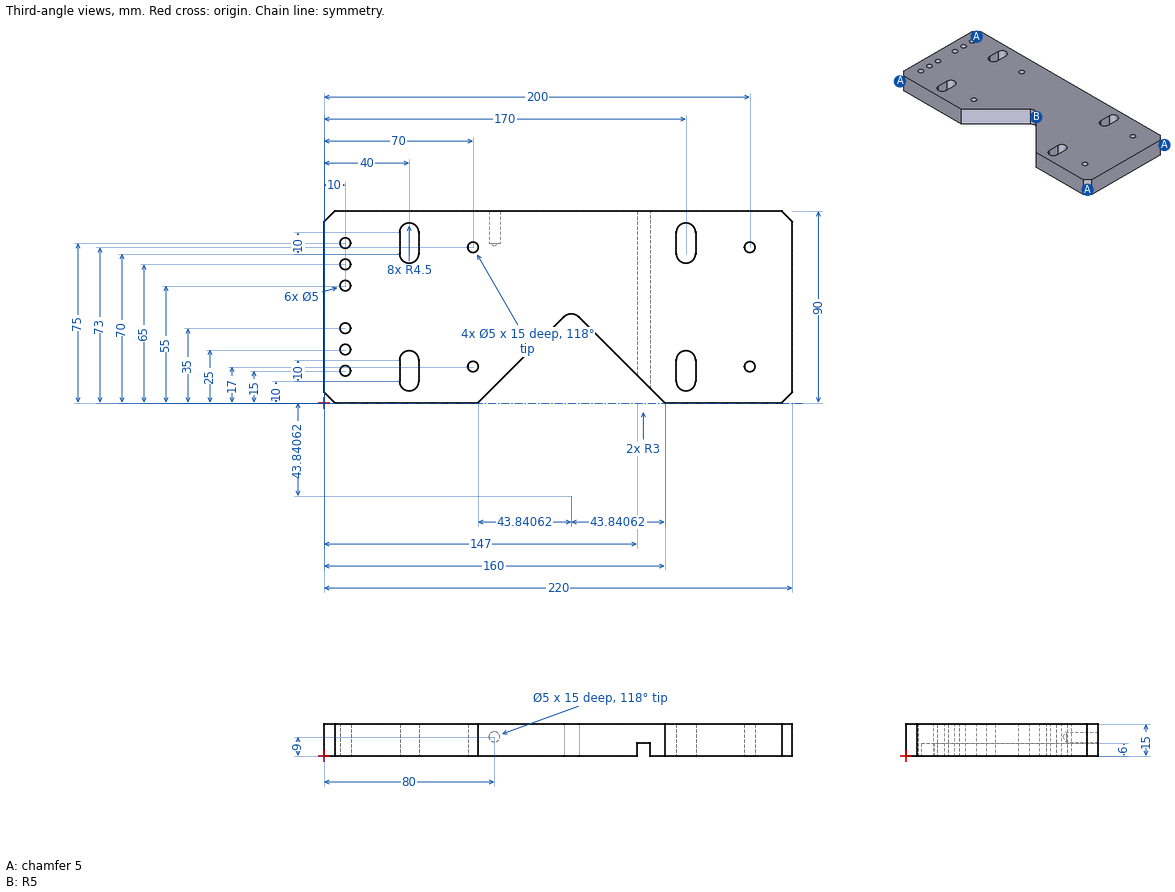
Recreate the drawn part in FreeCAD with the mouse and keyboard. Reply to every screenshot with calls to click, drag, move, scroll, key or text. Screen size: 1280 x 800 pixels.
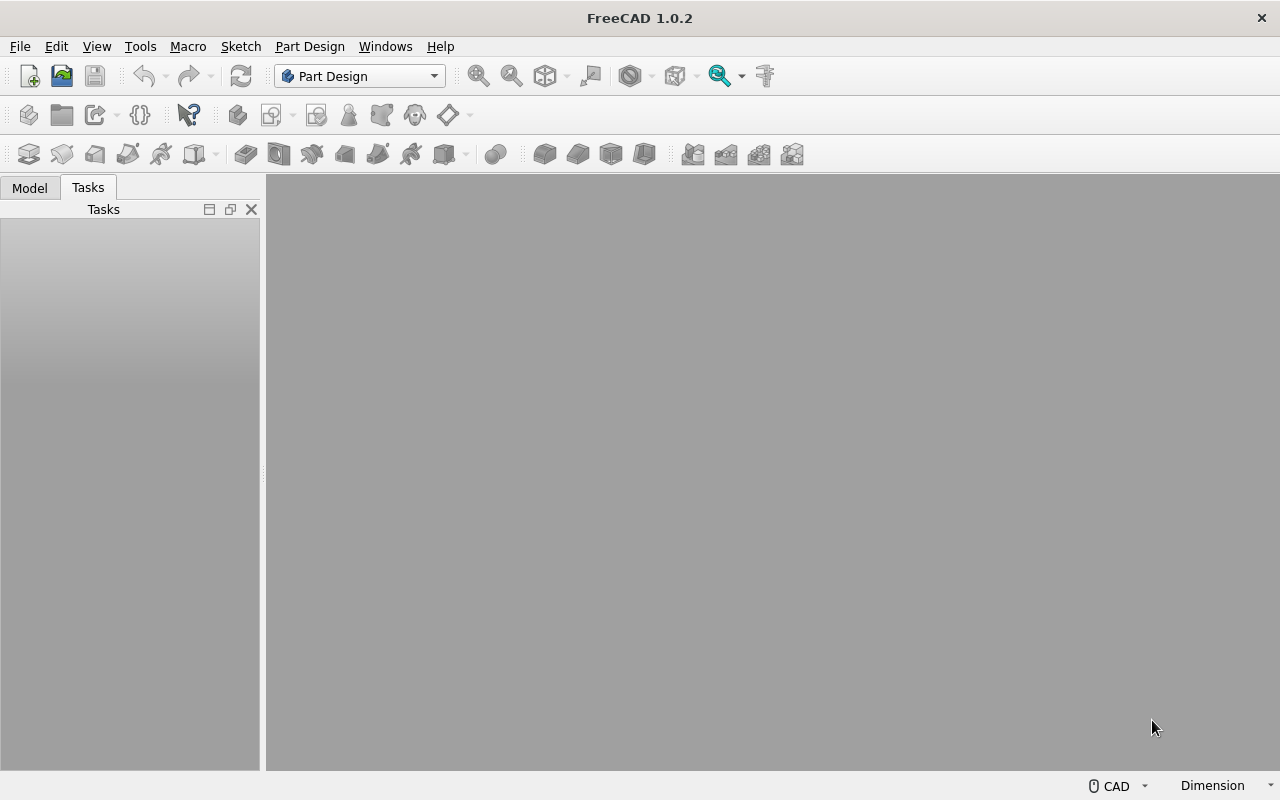
click(29, 76)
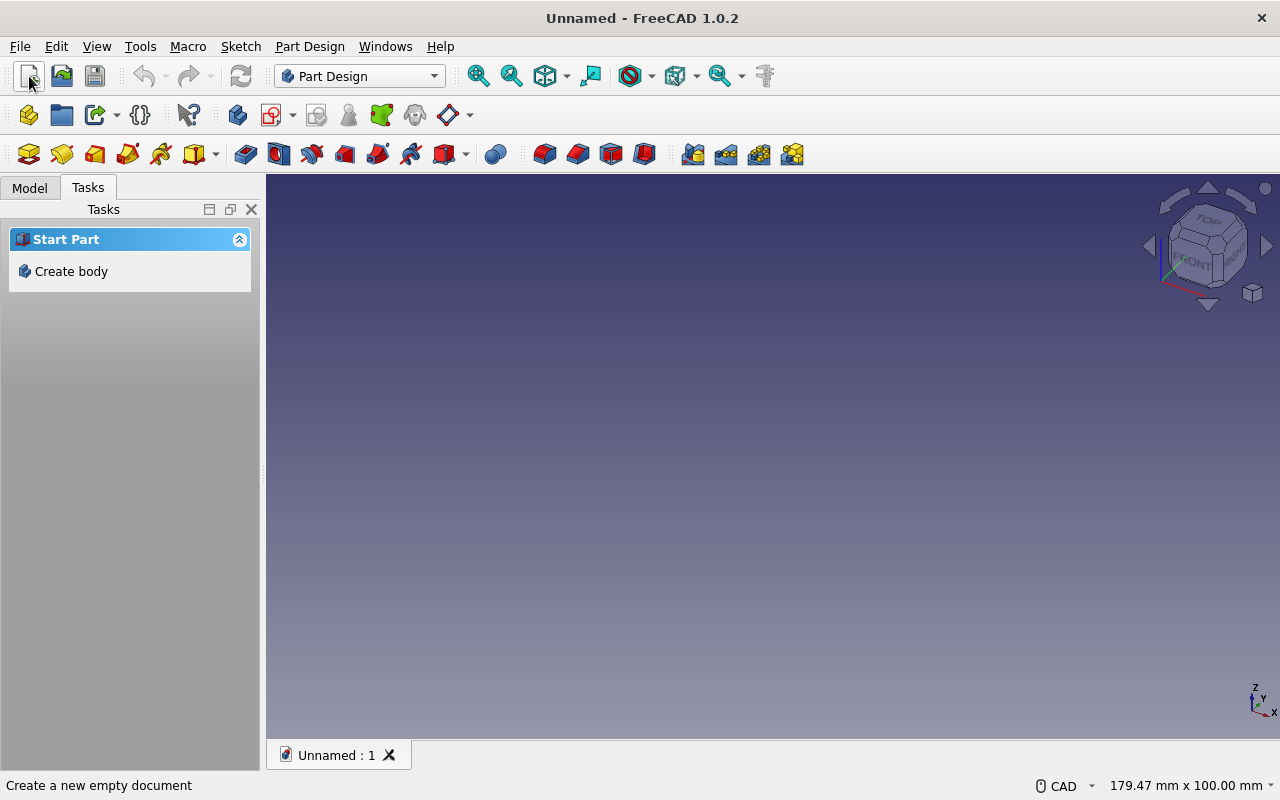
click(270, 116)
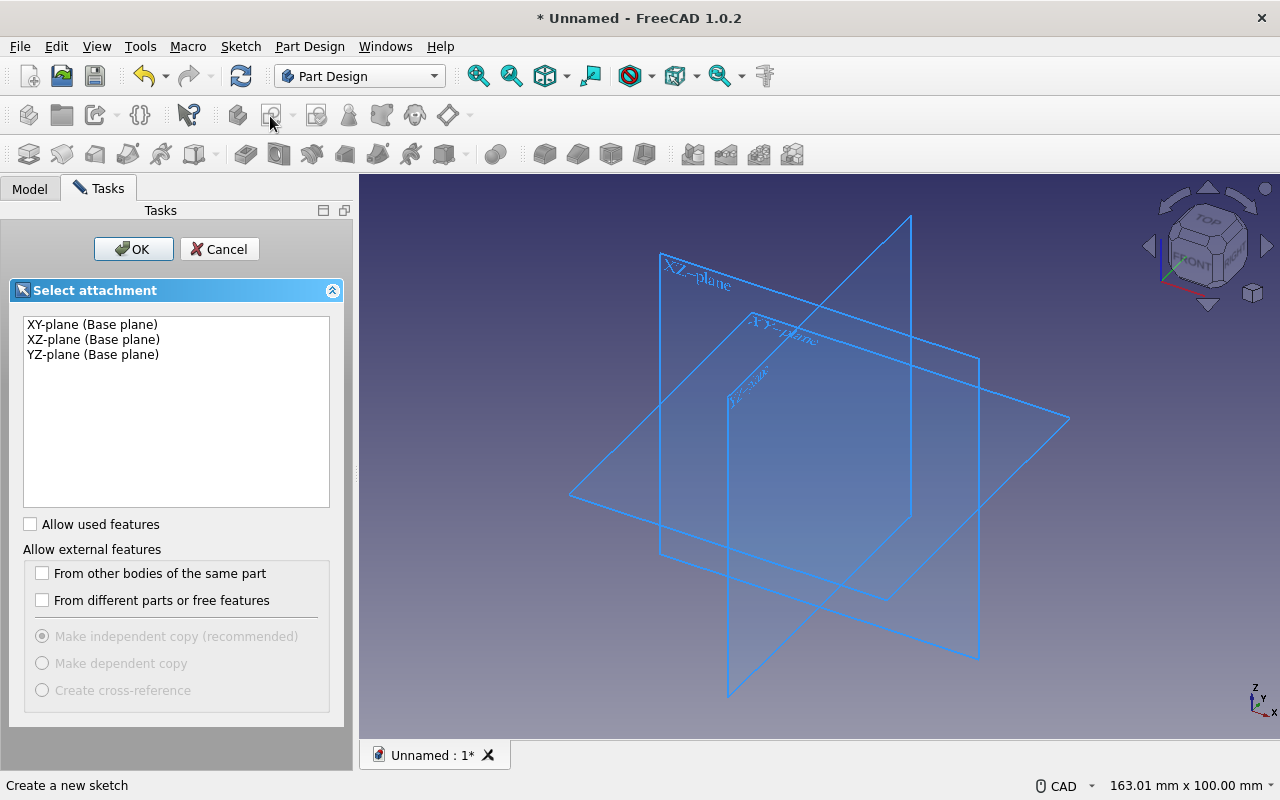
click(84, 324)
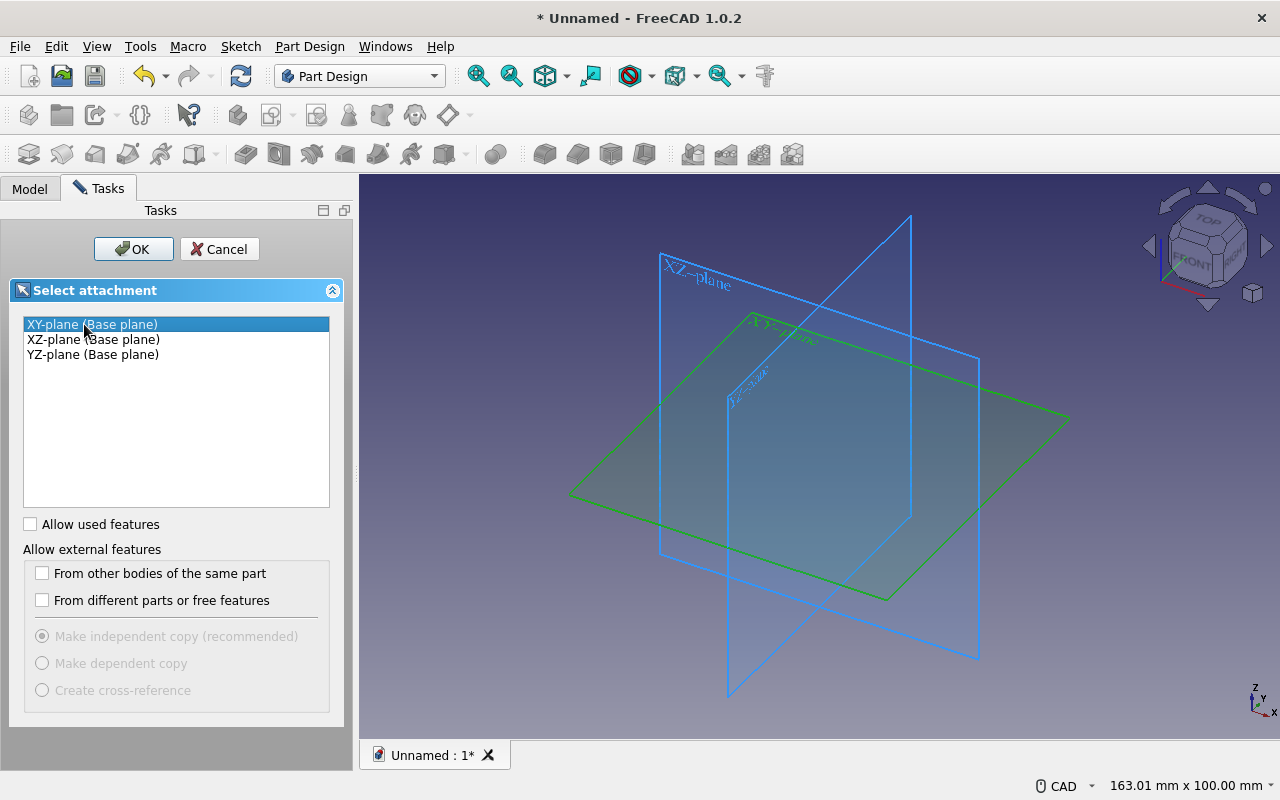
click(134, 249)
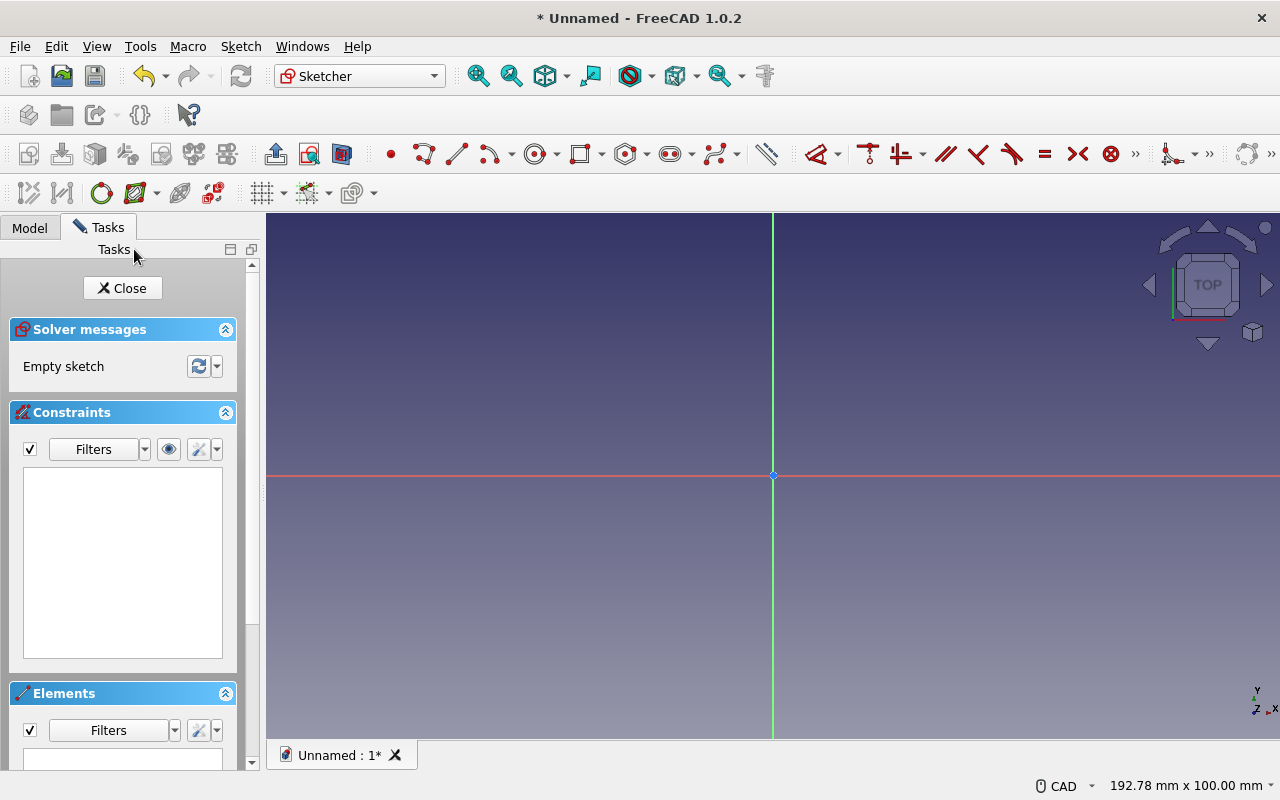
scroll(294, 669, down, 4)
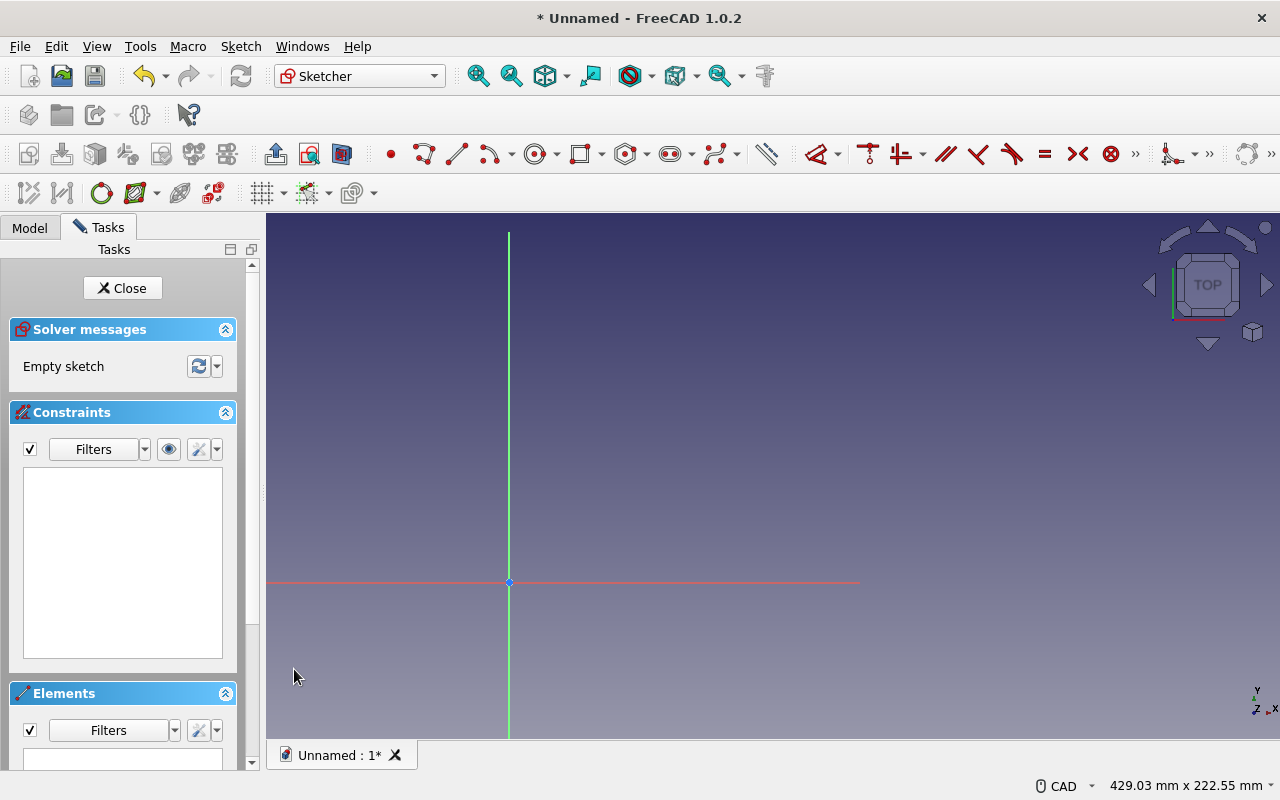
key(g)
key(r)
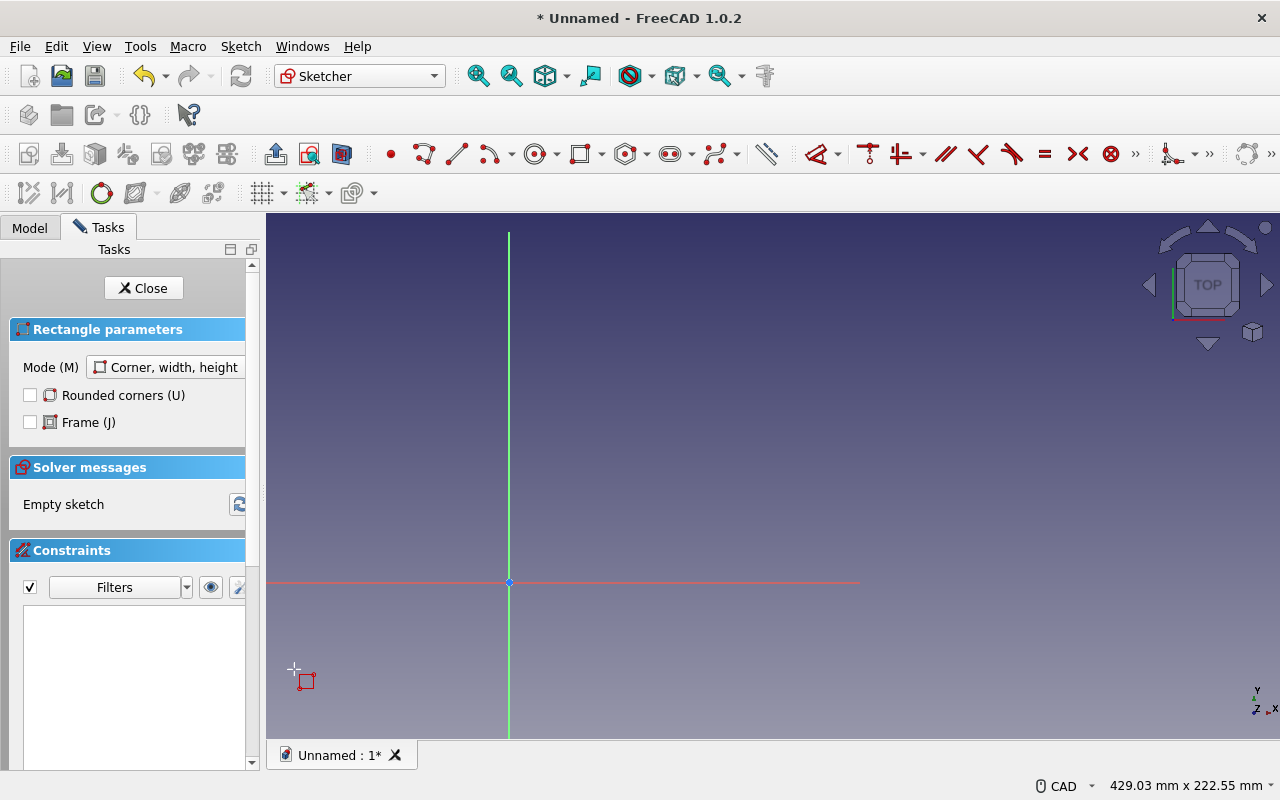
click(509, 583)
click(1029, 370)
key(Escape)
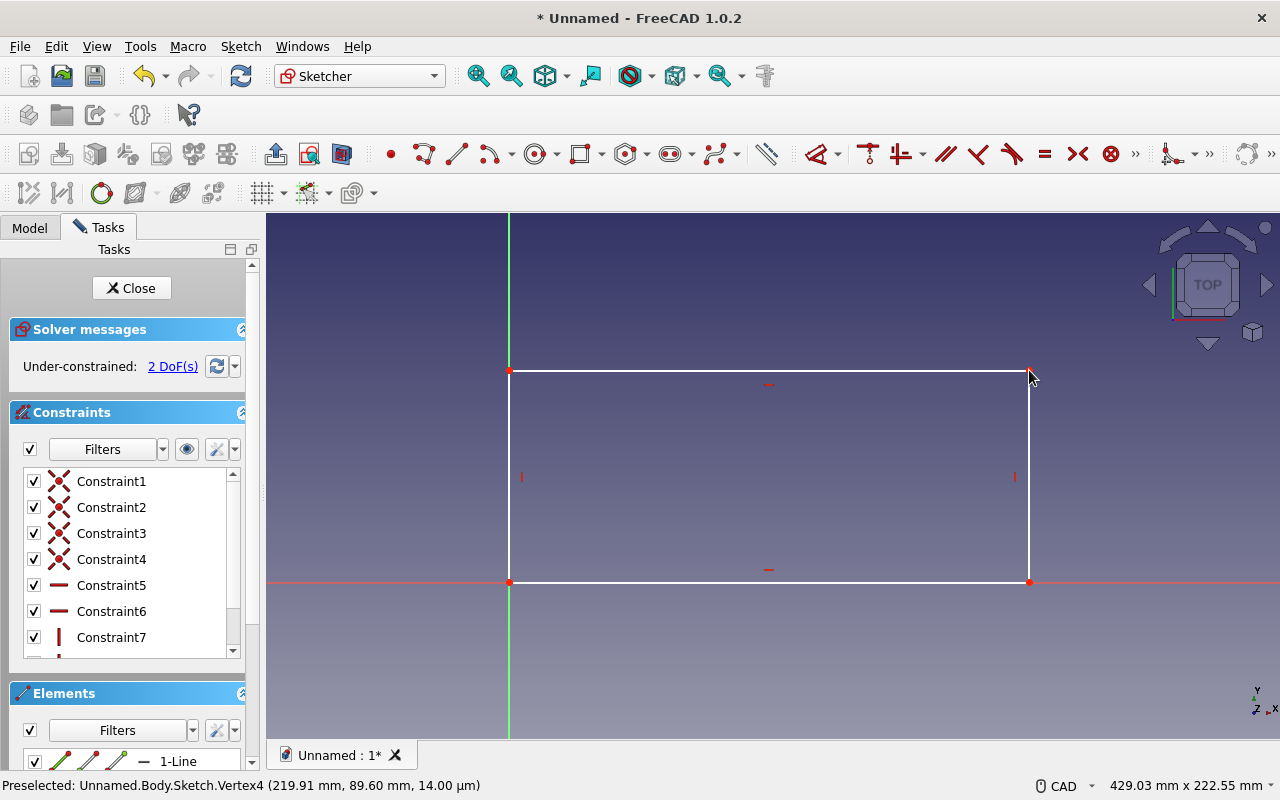
key(d)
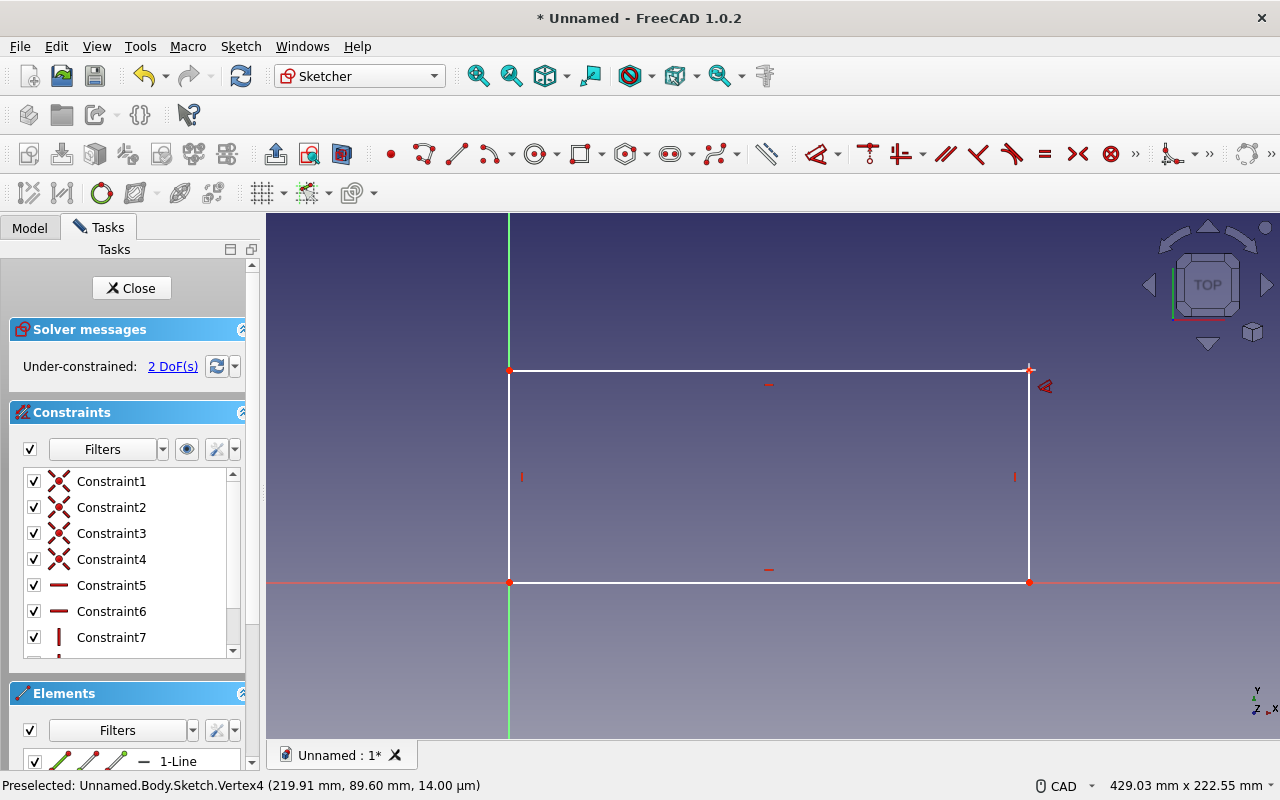
click(1029, 519)
click(1063, 477)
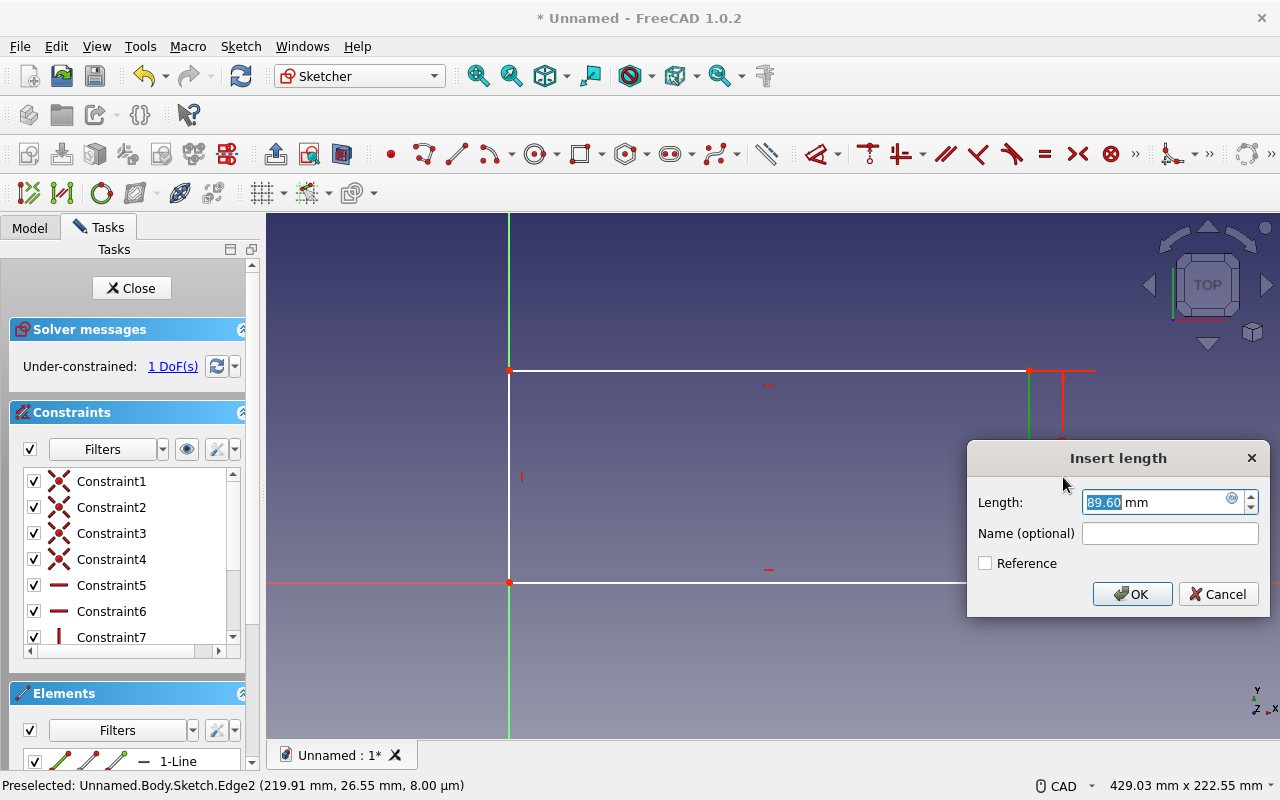
text(90)
key(Return)